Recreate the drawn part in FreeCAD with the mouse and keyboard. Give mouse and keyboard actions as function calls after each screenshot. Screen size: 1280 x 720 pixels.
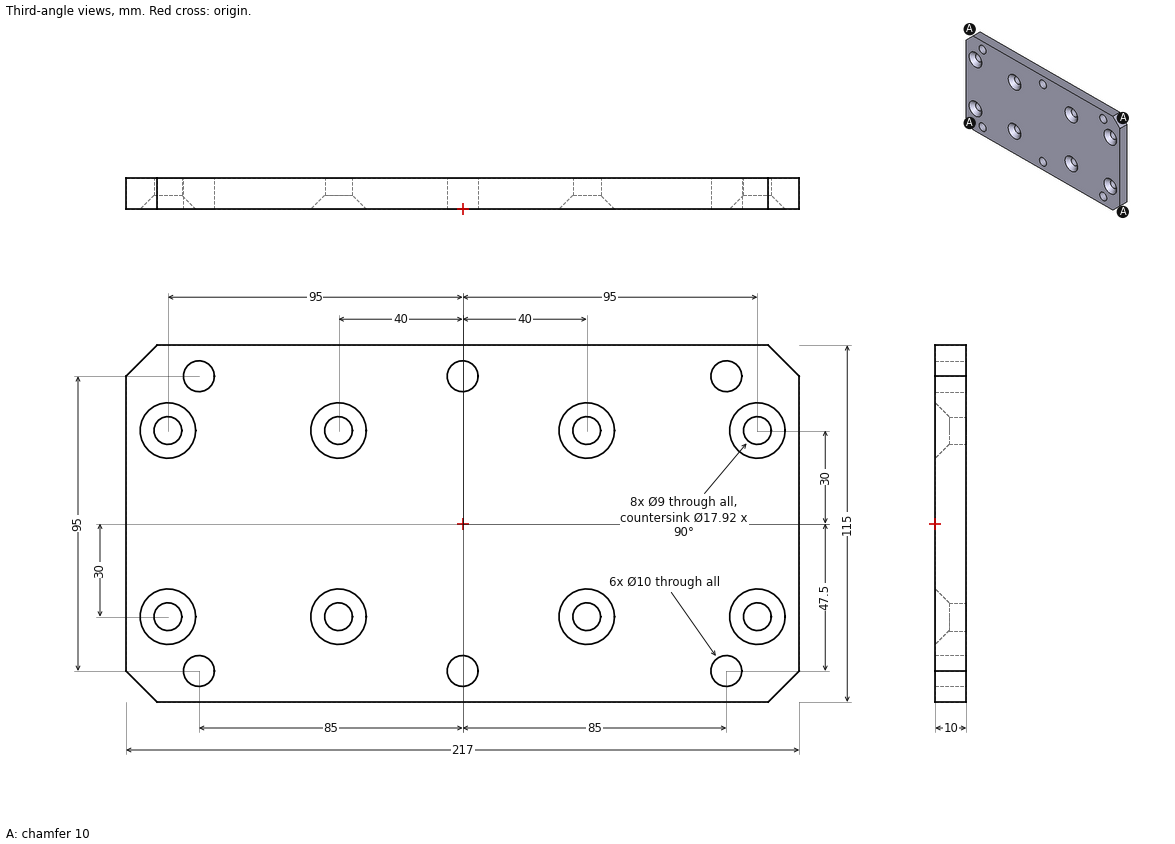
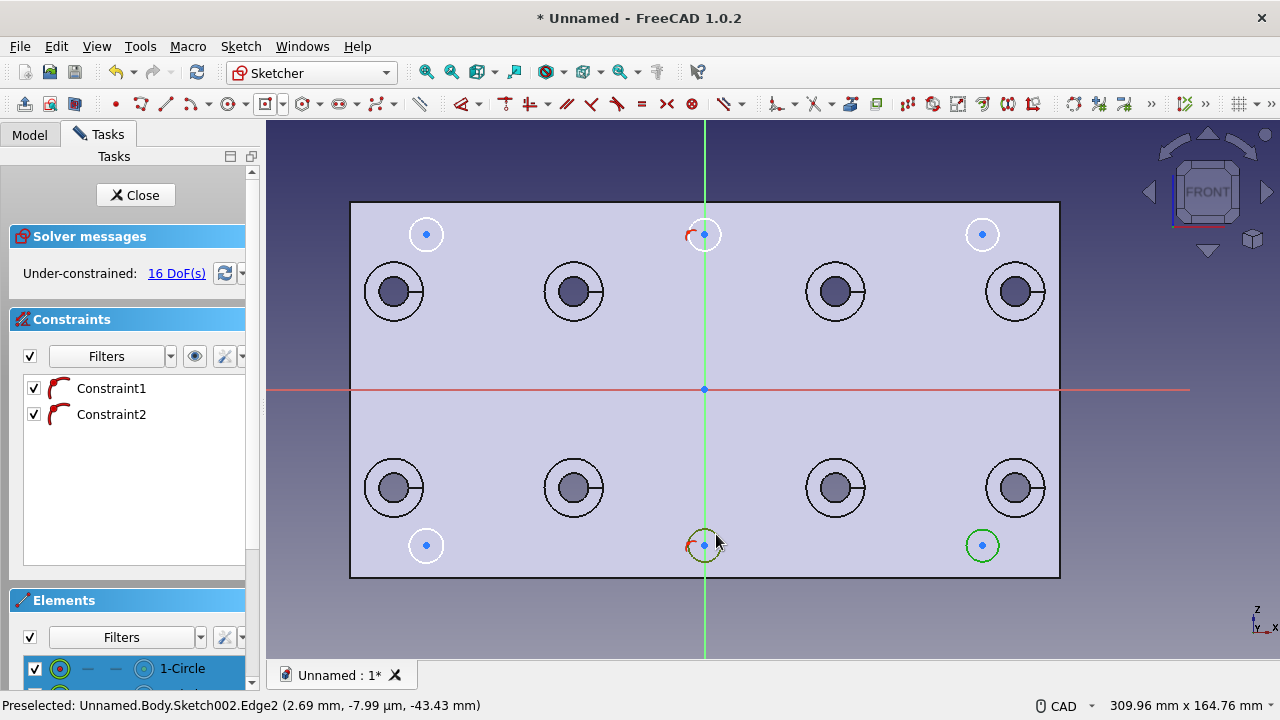
click(438, 534)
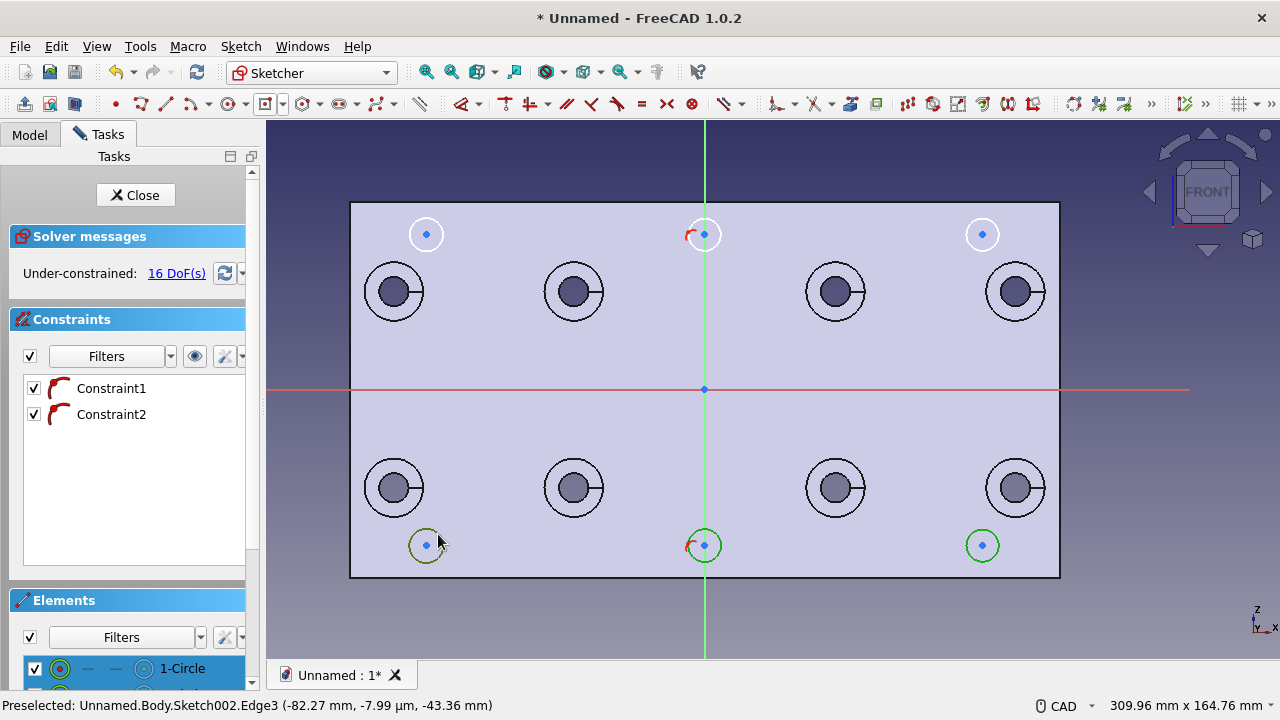
click(438, 223)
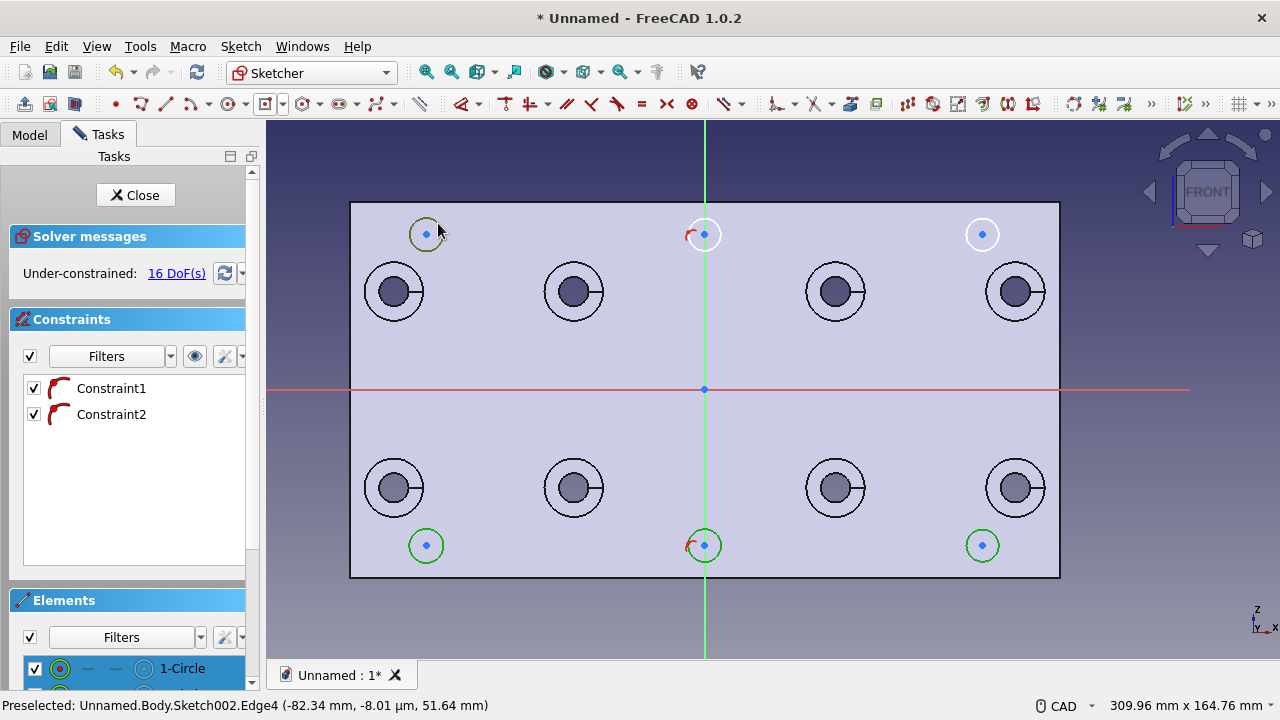
click(716, 223)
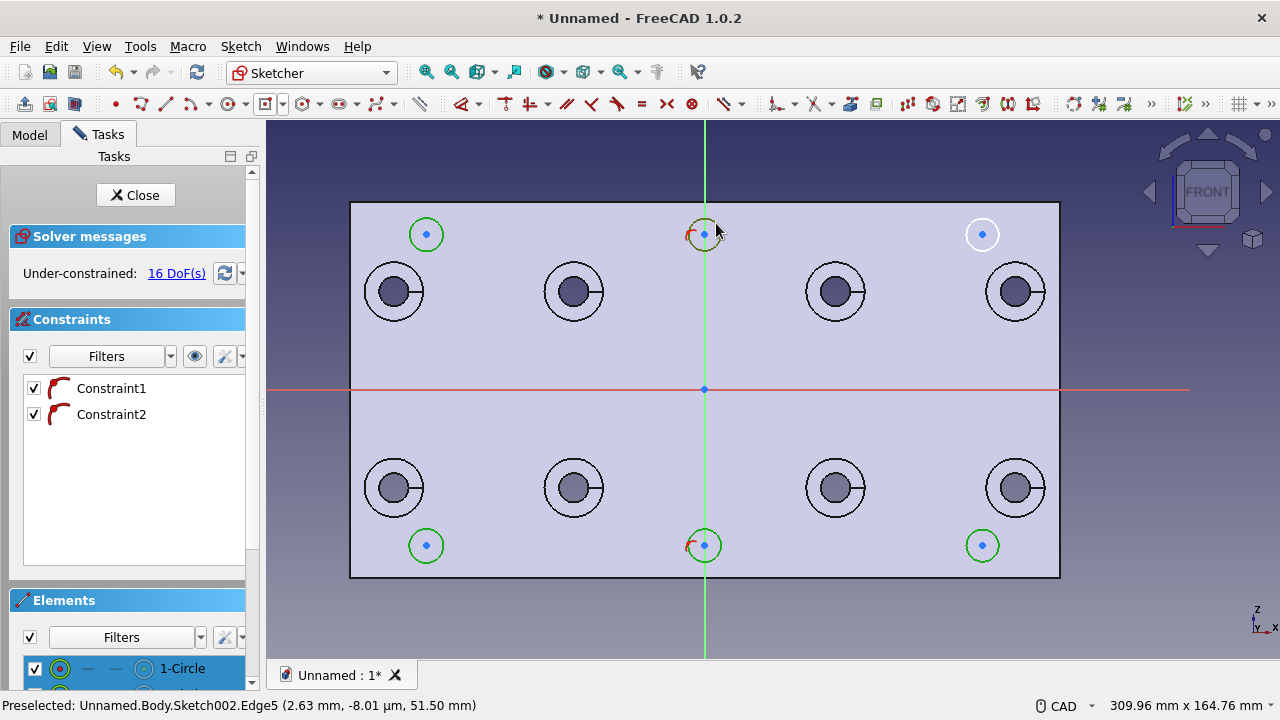
click(994, 223)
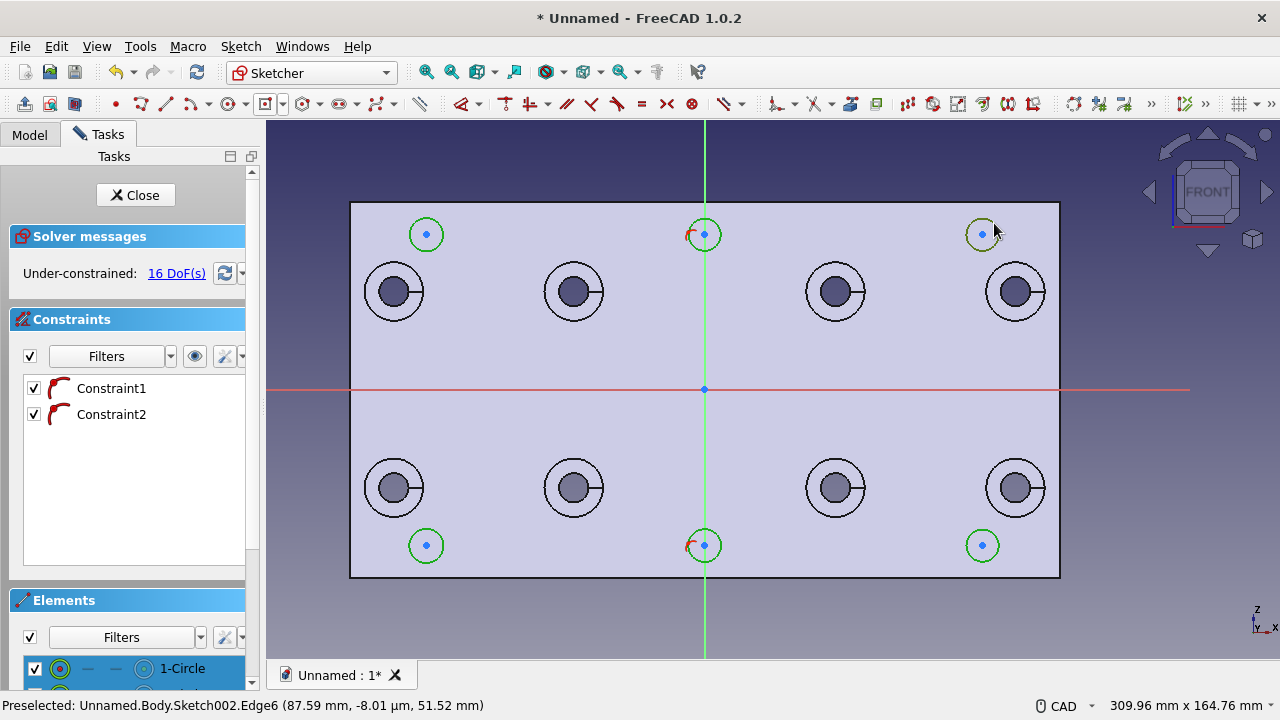
click(642, 104)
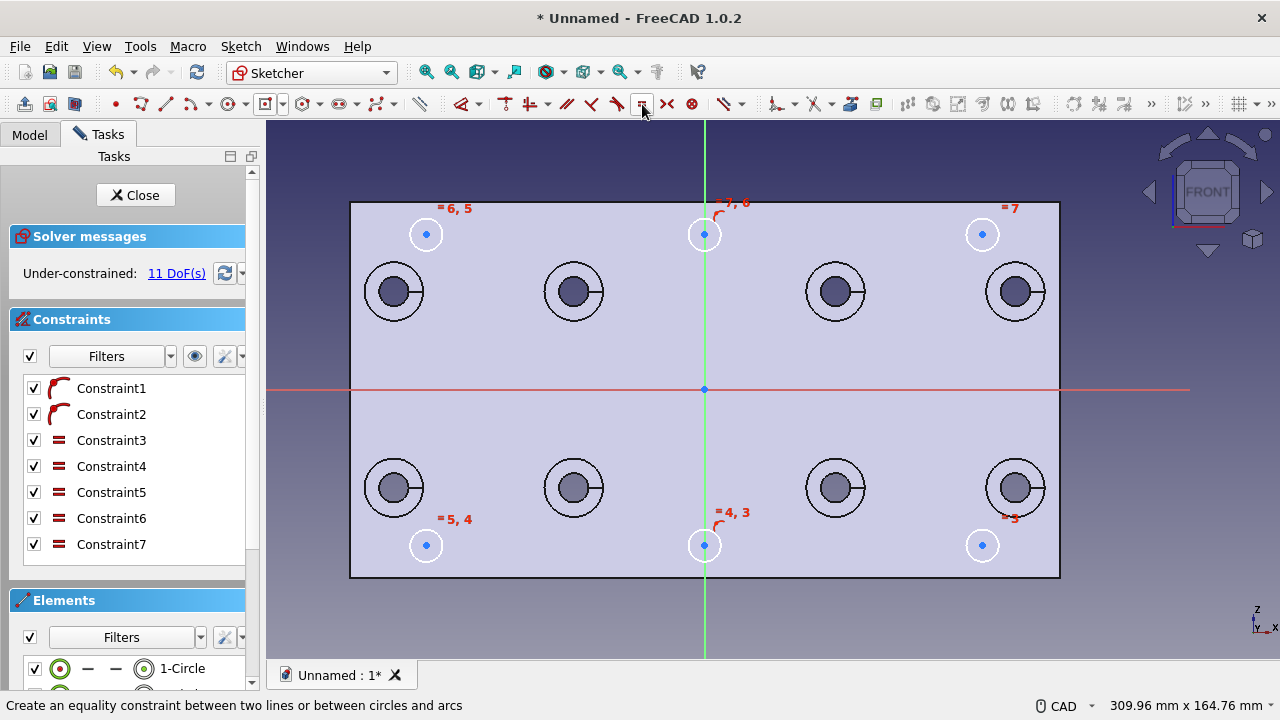
click(460, 104)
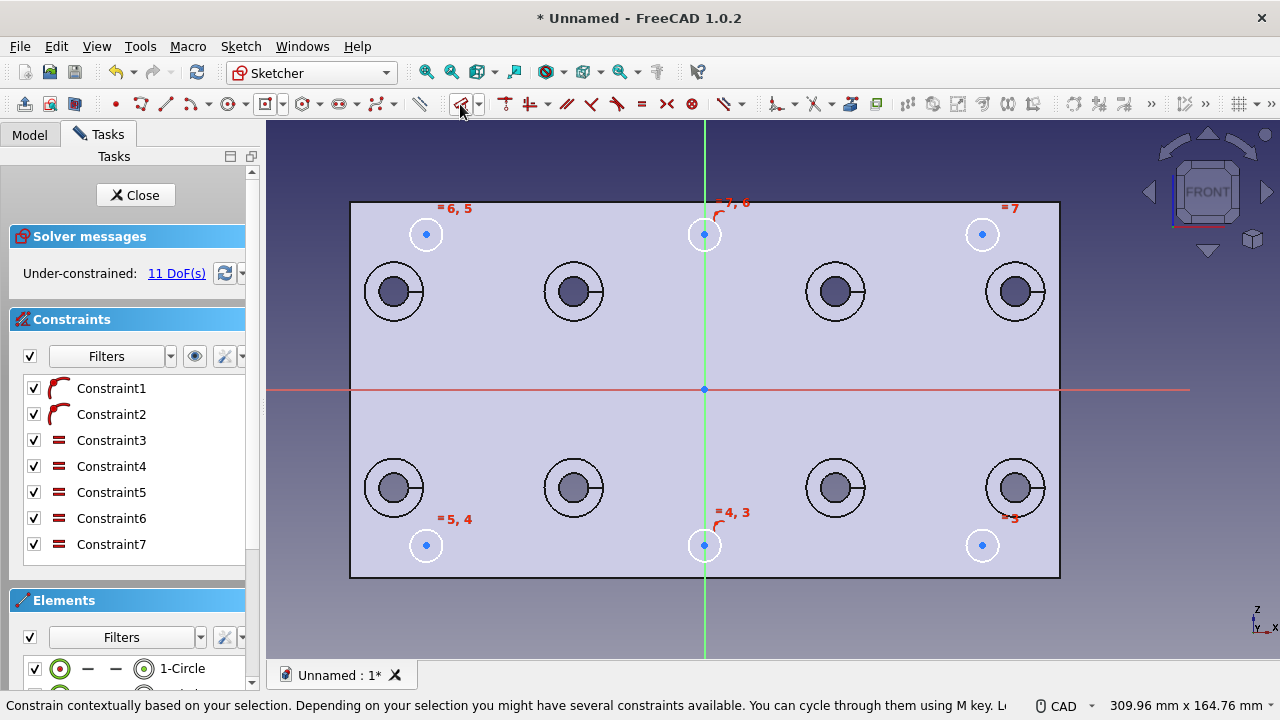
click(994, 534)
click(1016, 511)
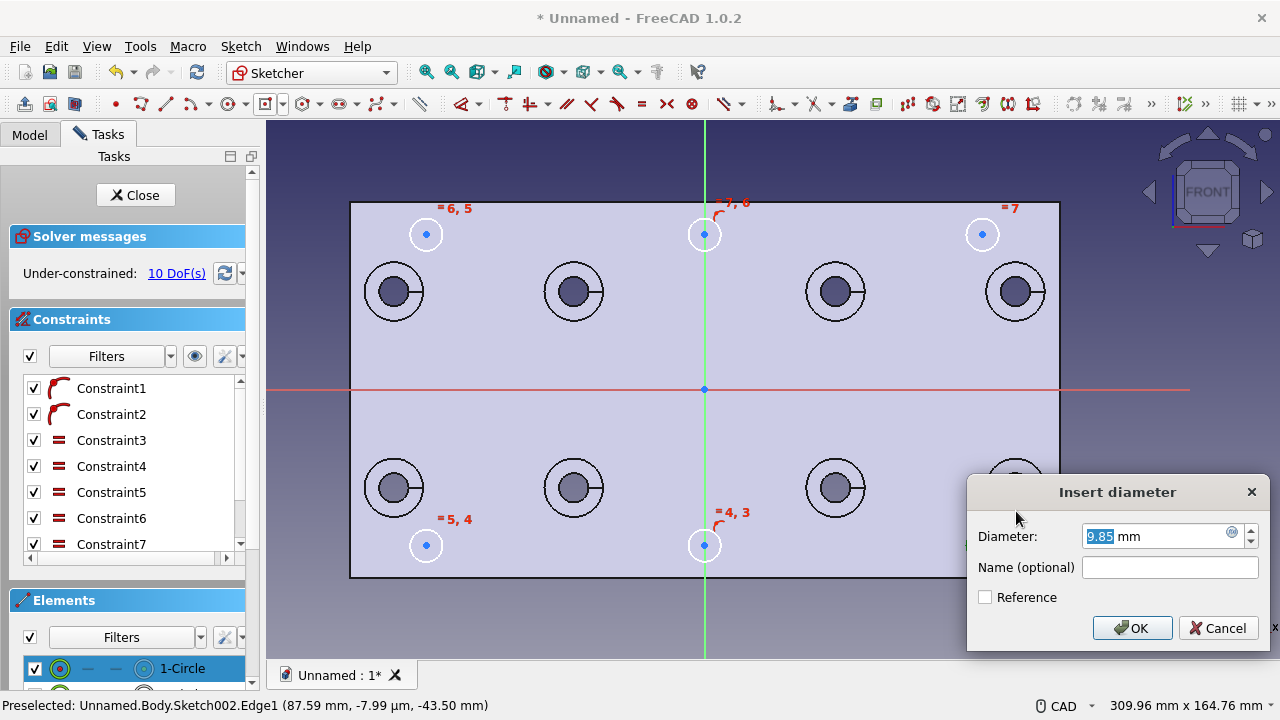
text(10)
key(Return)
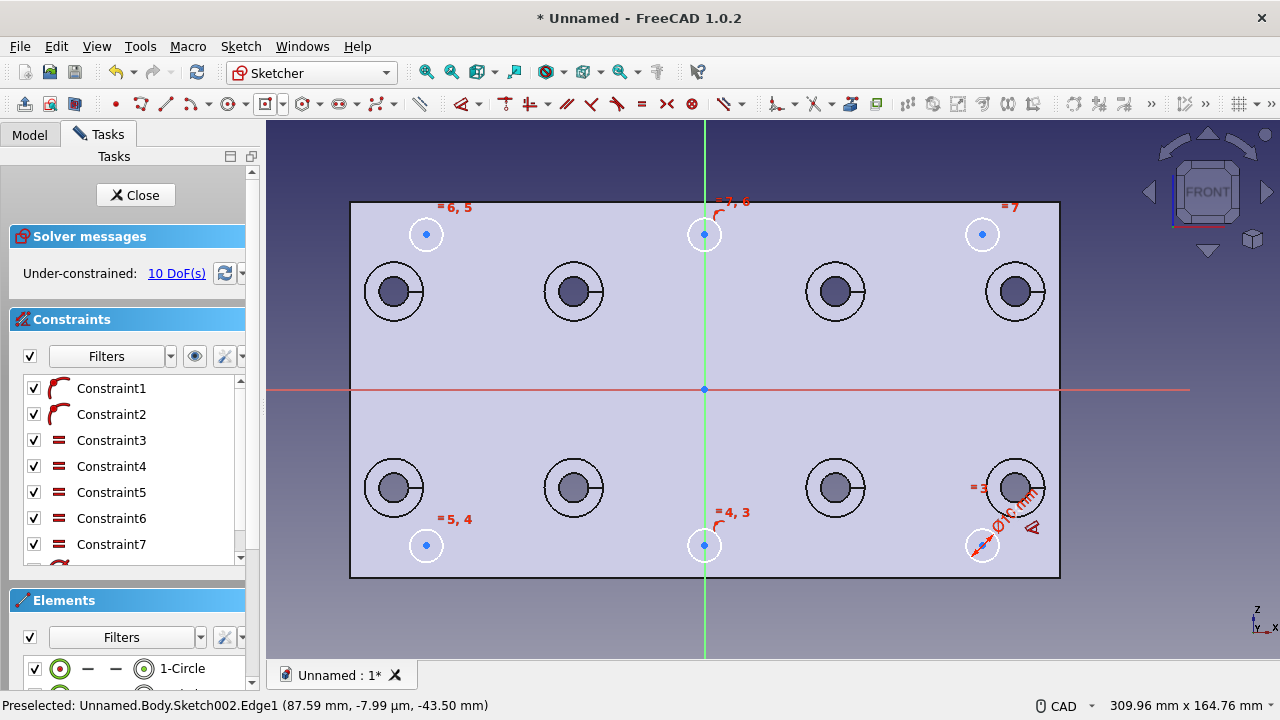
click(983, 546)
click(844, 580)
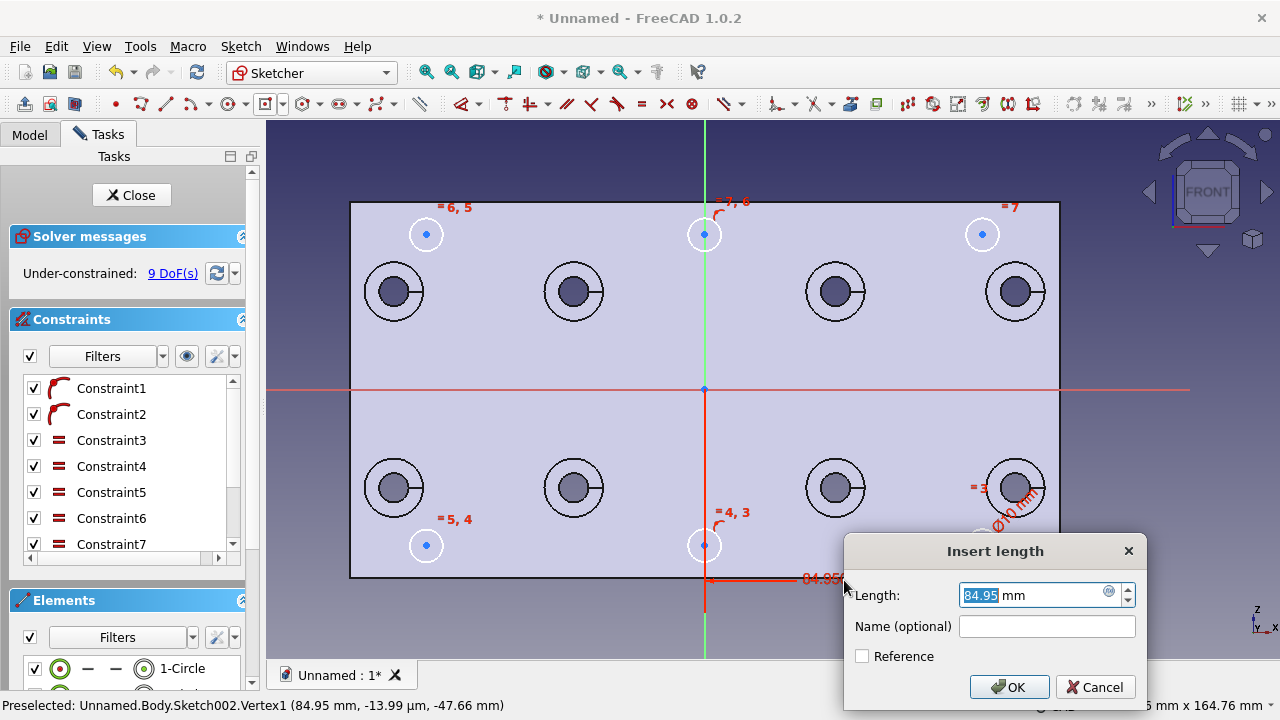
text(85)
key(Return)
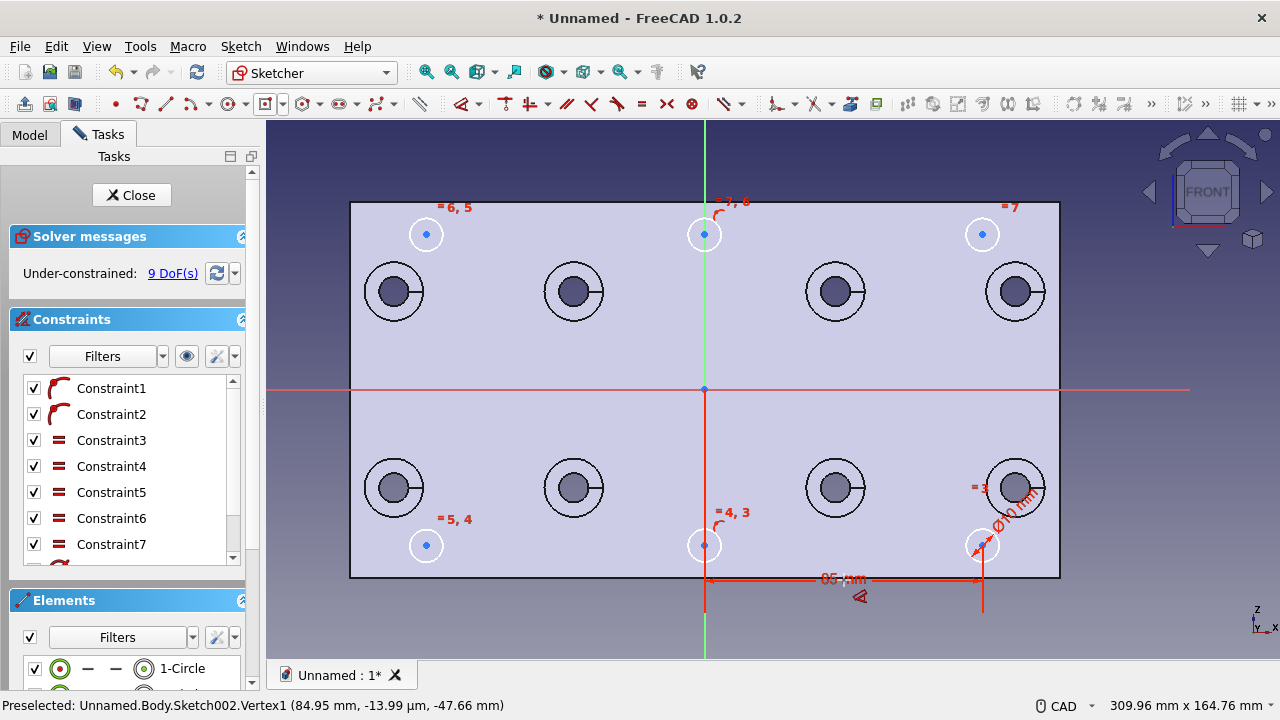
click(426, 546)
click(566, 580)